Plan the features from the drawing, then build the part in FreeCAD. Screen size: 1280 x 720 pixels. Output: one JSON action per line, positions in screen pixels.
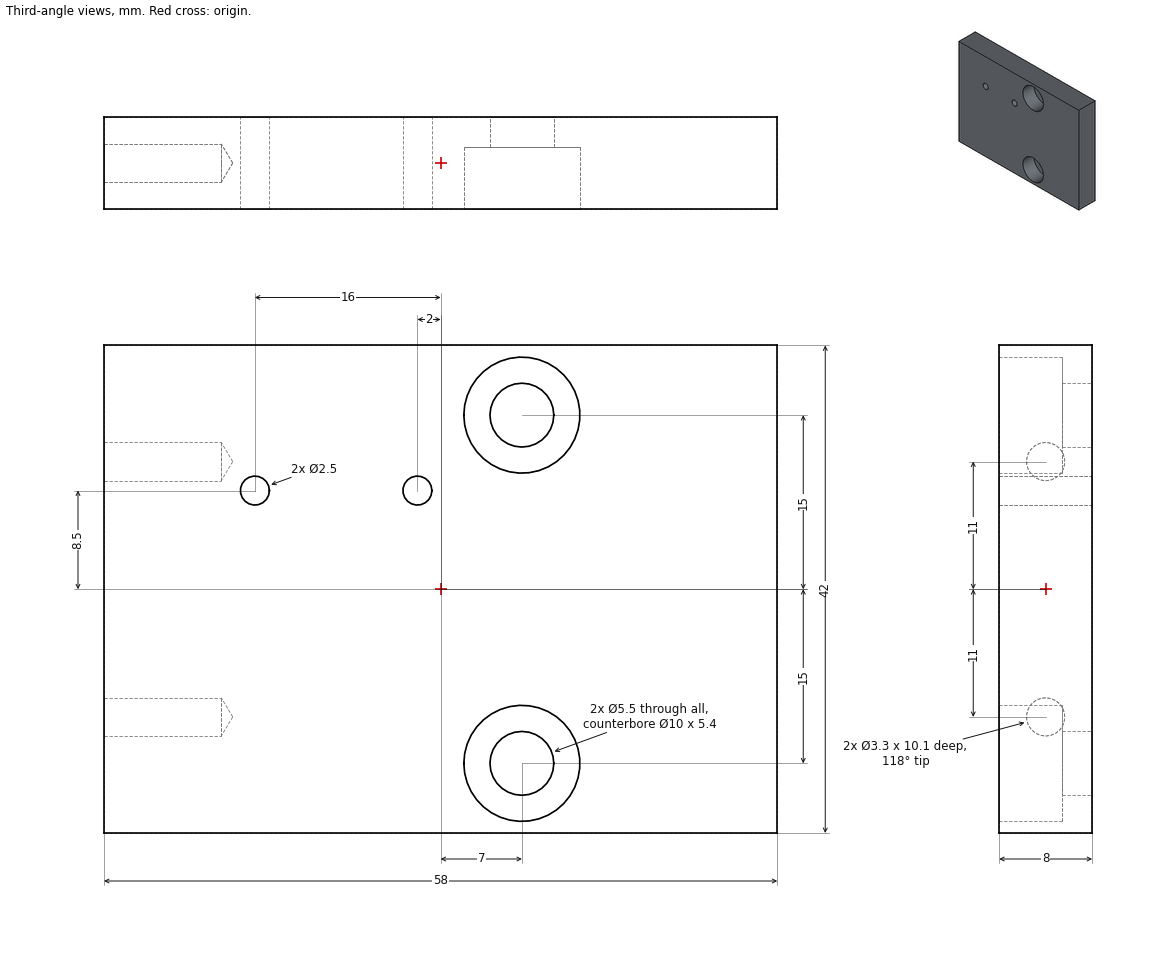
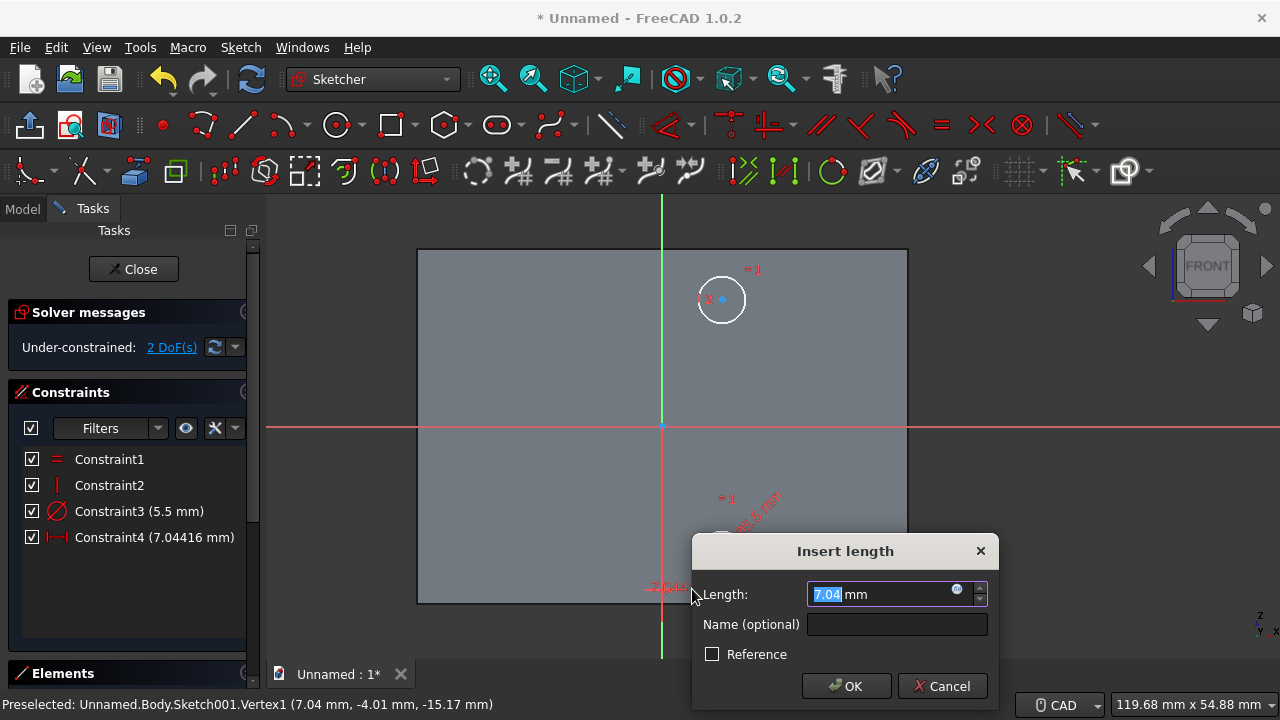
{"action": "type", "text": "7"}
{"action": "key", "text": "Return"}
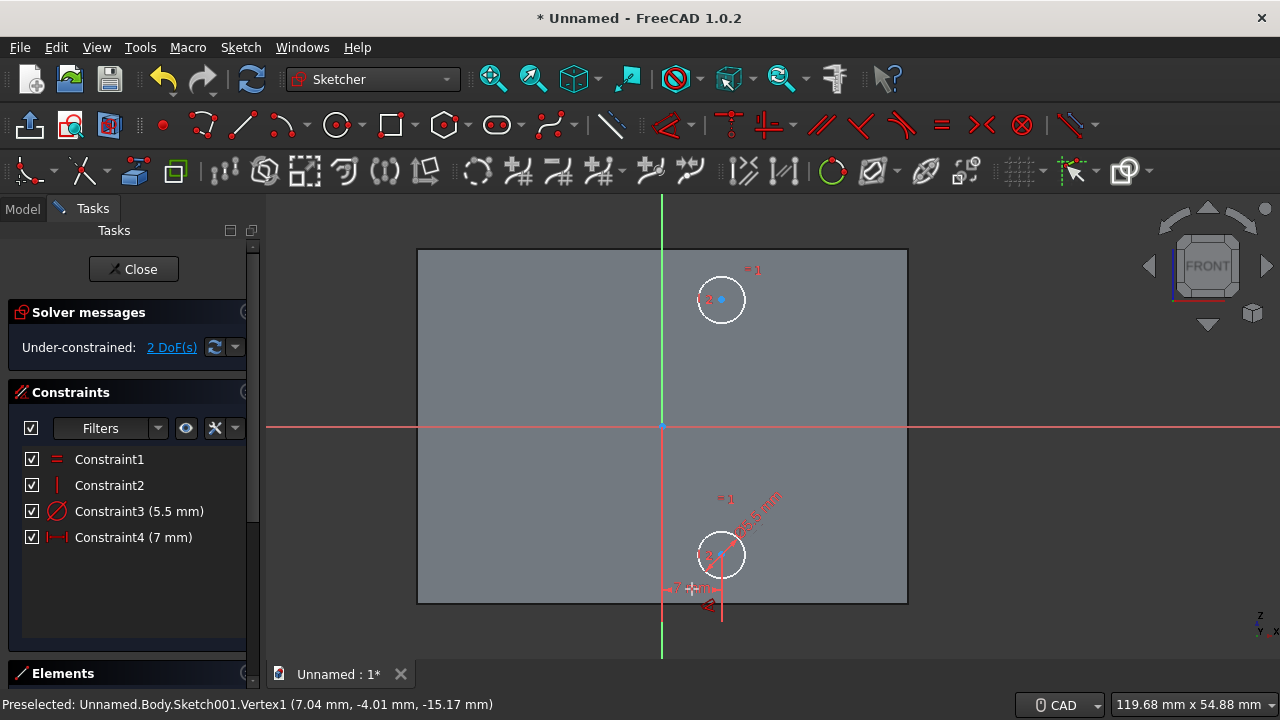
{"action": "left_click", "coordinate": [722, 555]}
{"action": "left_click", "coordinate": [628, 491]}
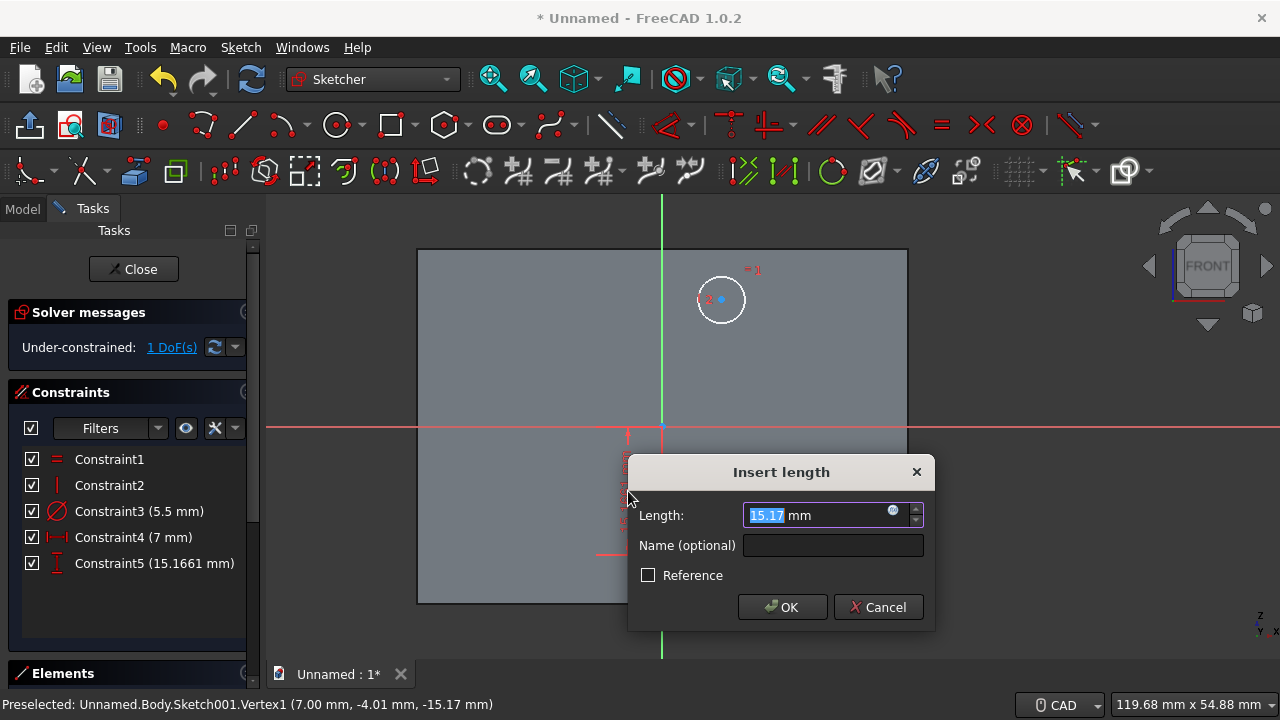
{"action": "type", "text": "15"}
{"action": "key", "text": "Return"}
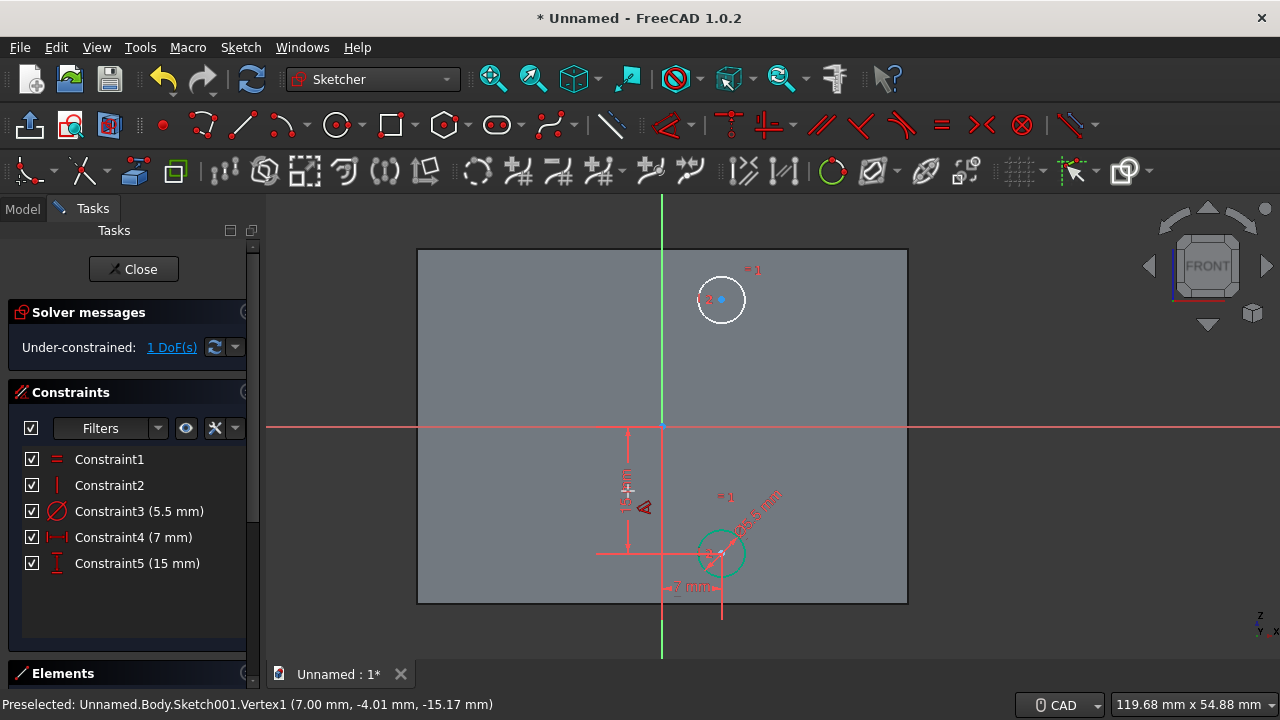
{"action": "left_click", "coordinate": [722, 300]}
{"action": "left_click", "coordinate": [628, 363]}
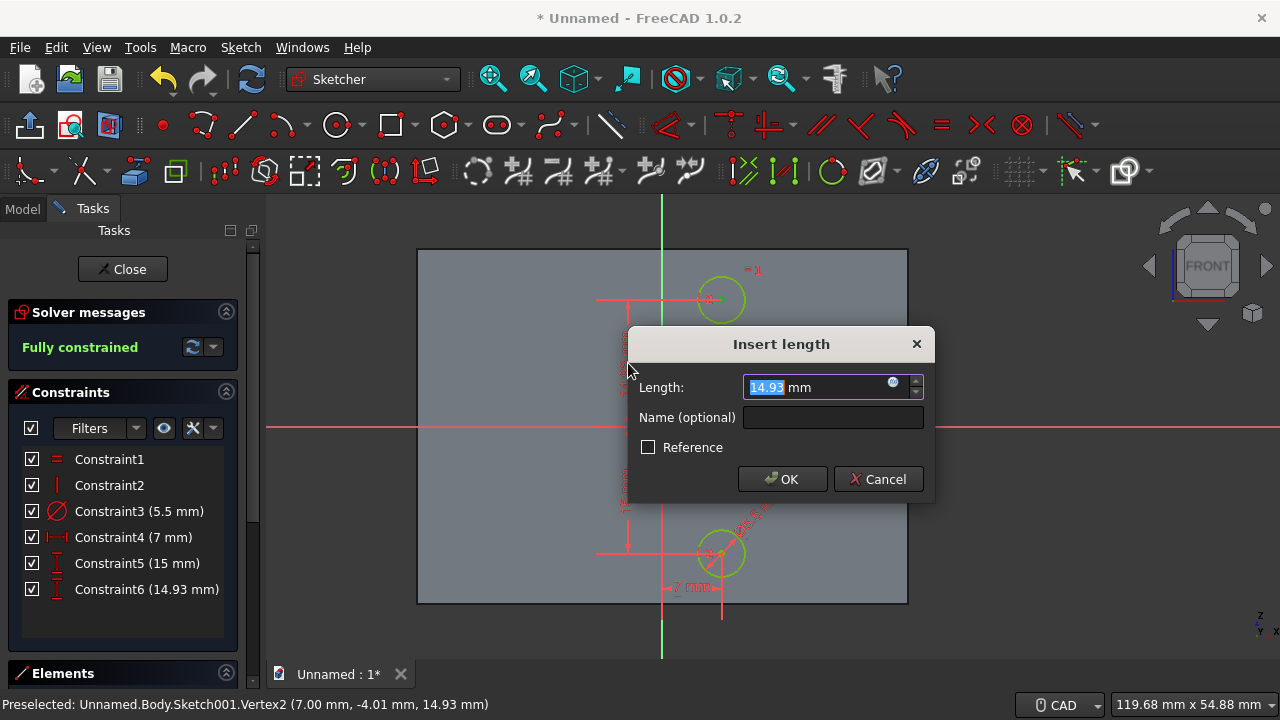
{"action": "type", "text": "15"}
{"action": "key", "text": "Return"}
{"action": "key", "text": "Escape"}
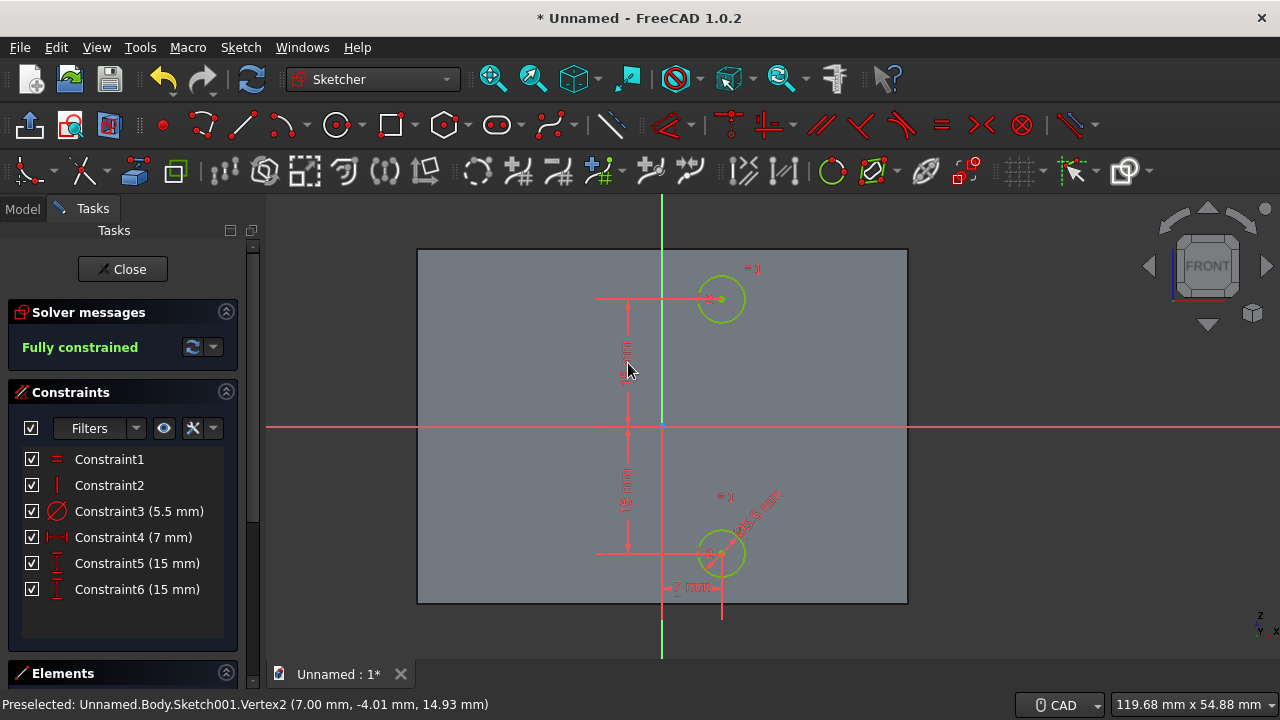
{"action": "left_click", "coordinate": [123, 269]}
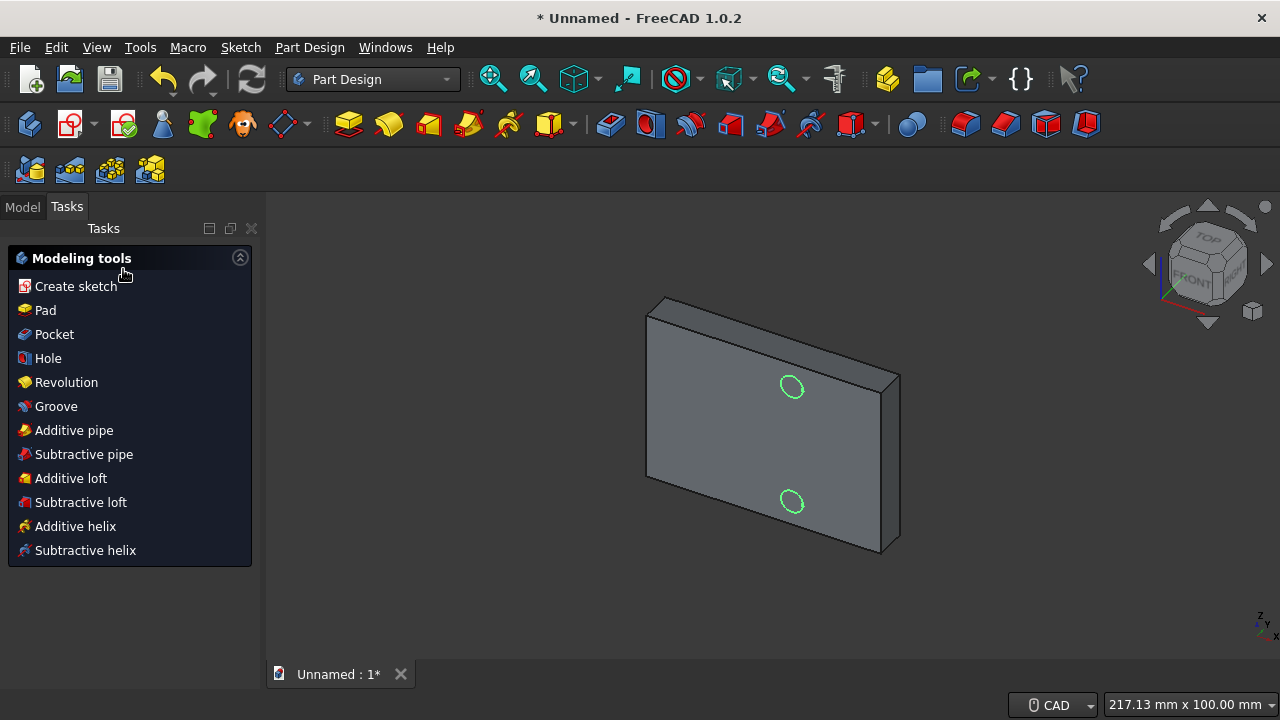
{"action": "left_click", "coordinate": [652, 124]}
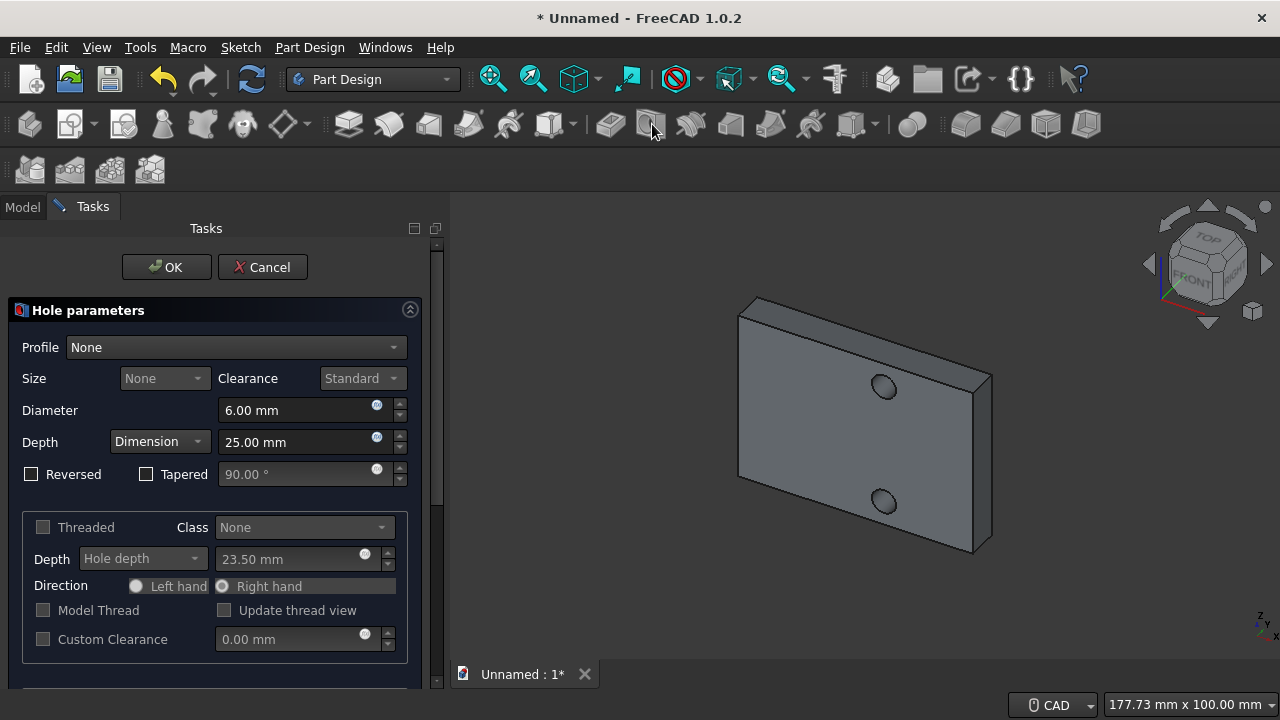
{"action": "triple_click", "coordinate": [305, 410]}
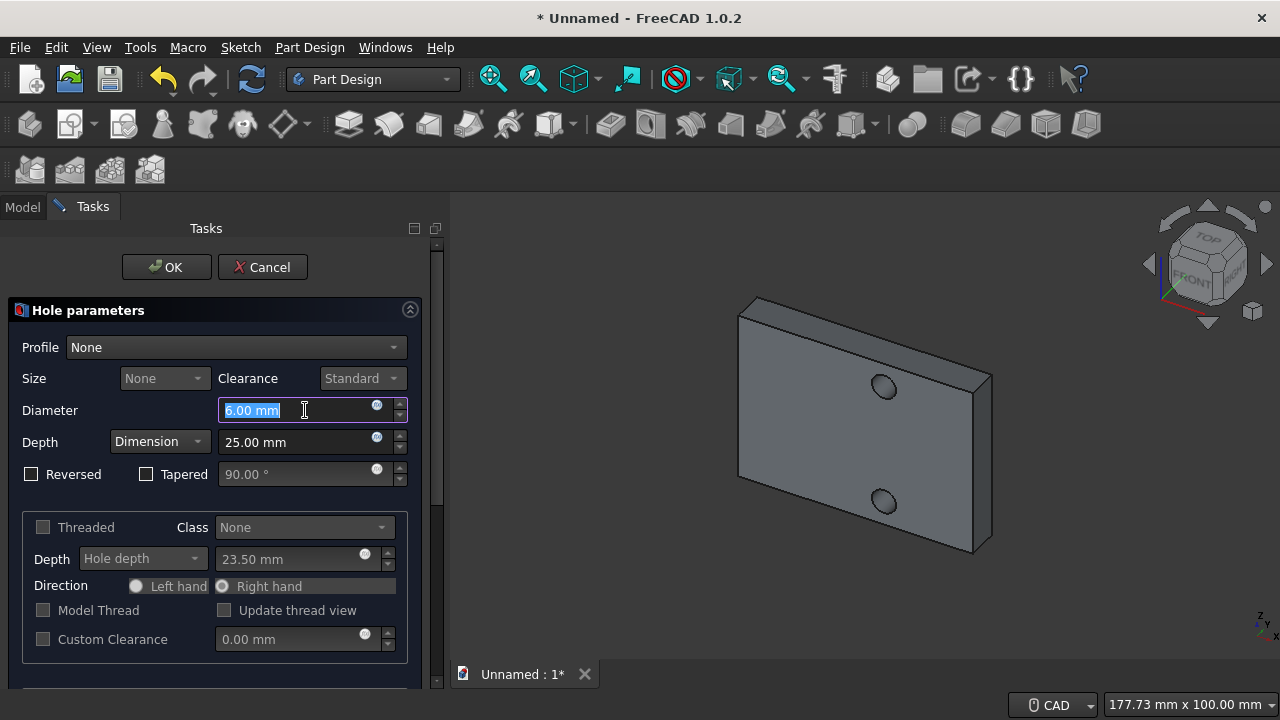
{"action": "type", "text": "5.5"}
{"action": "key", "text": "Tab"}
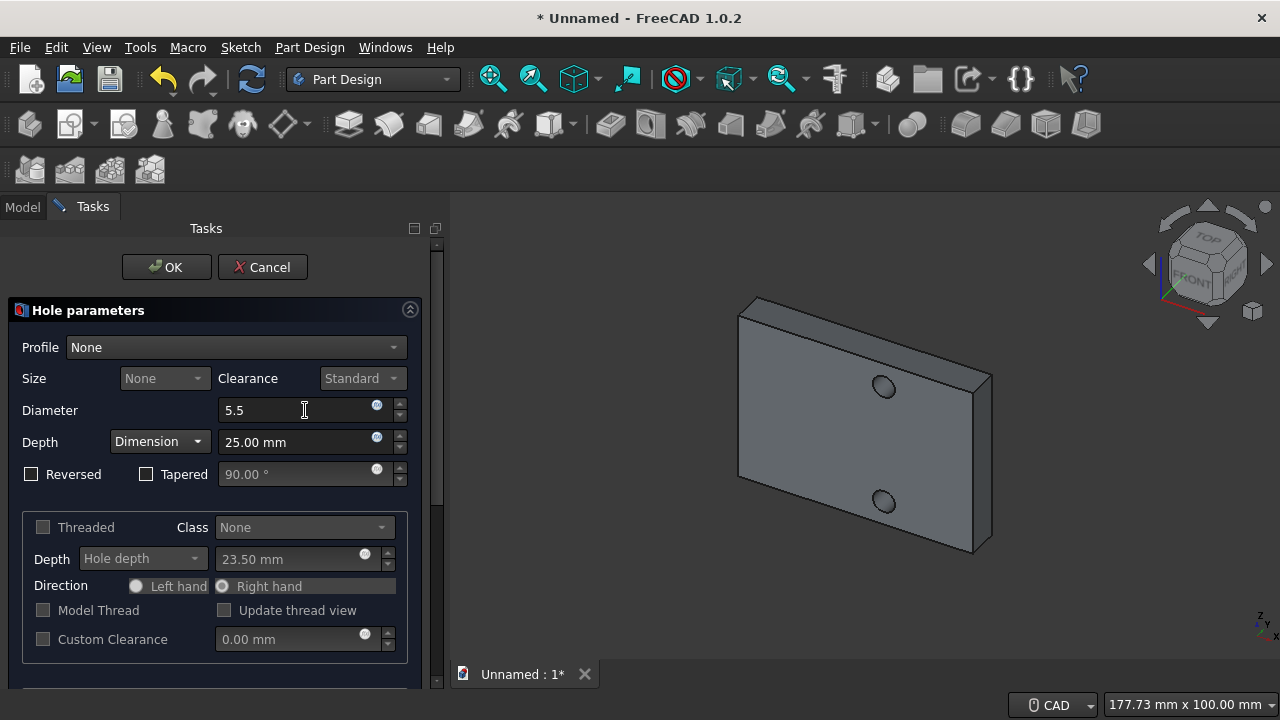
{"action": "left_click", "coordinate": [161, 442]}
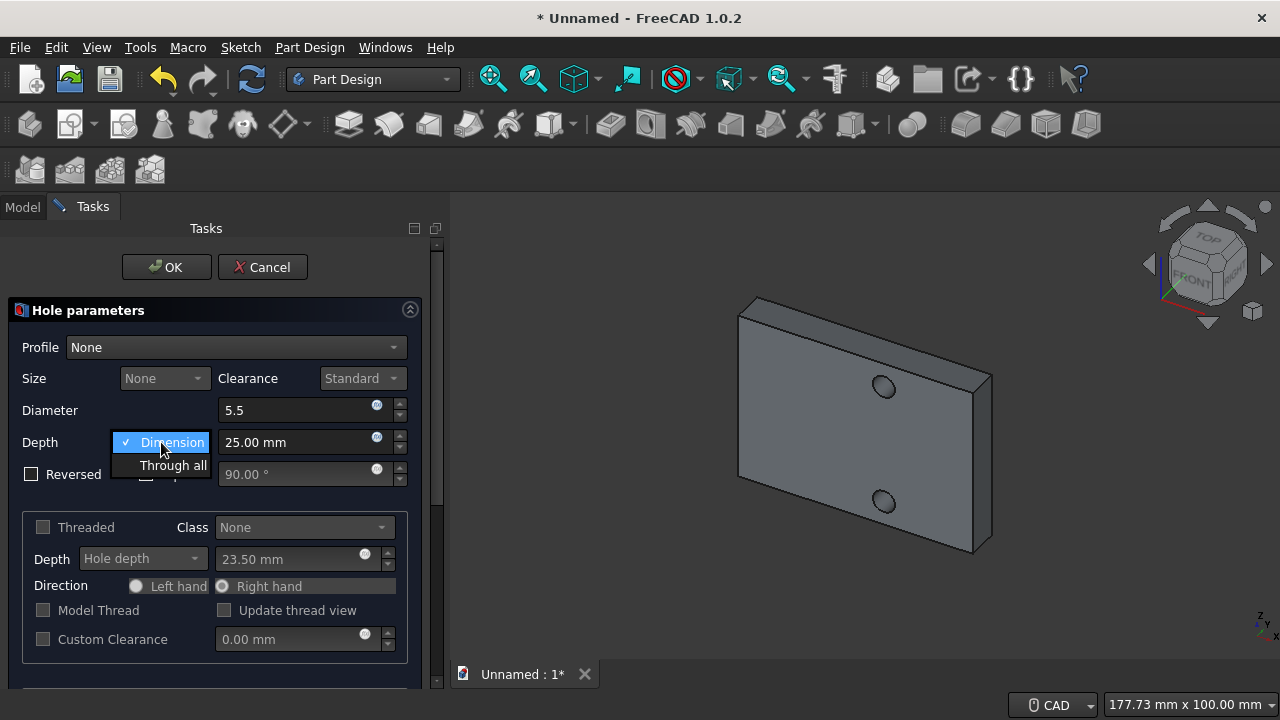
{"action": "left_click", "coordinate": [160, 466]}